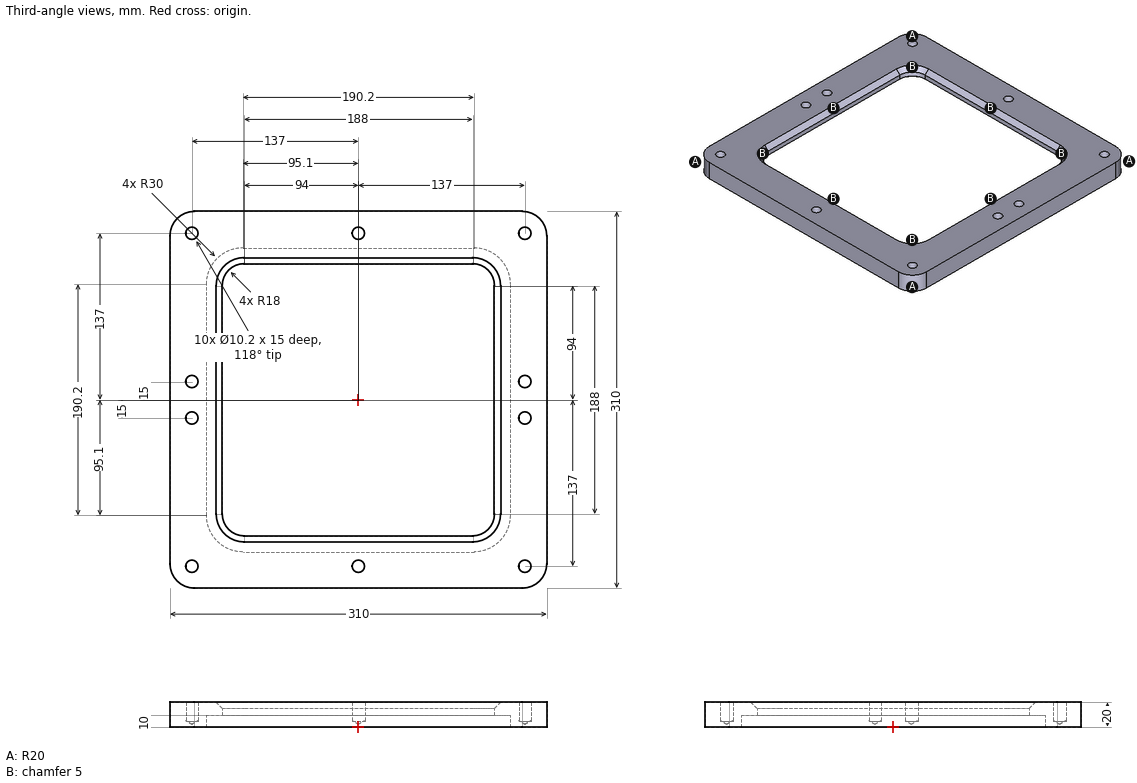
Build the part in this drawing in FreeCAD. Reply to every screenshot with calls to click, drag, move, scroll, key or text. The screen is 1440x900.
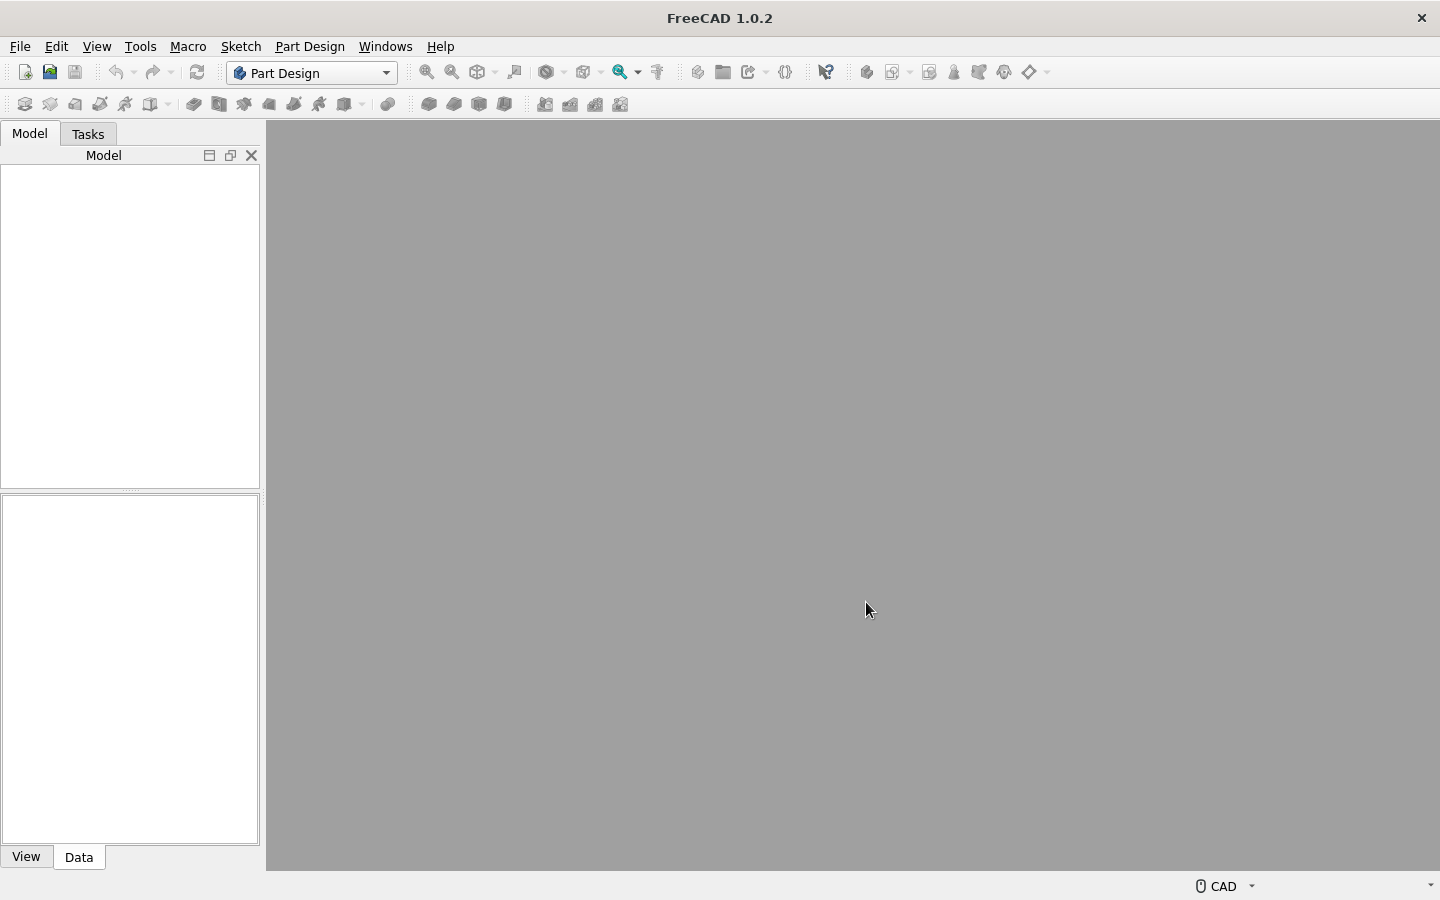
click(25, 72)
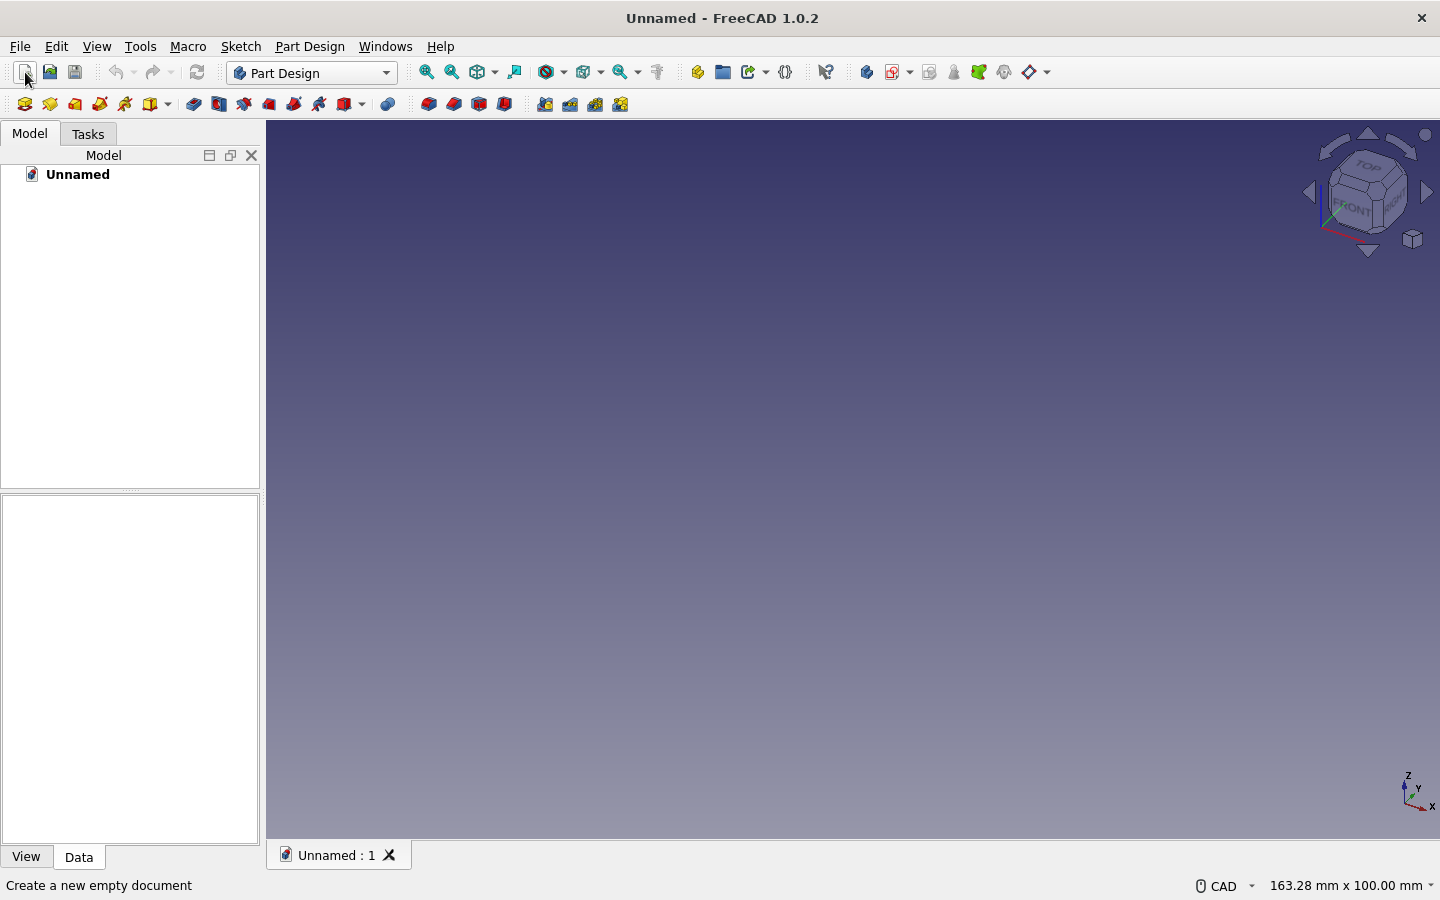
click(892, 72)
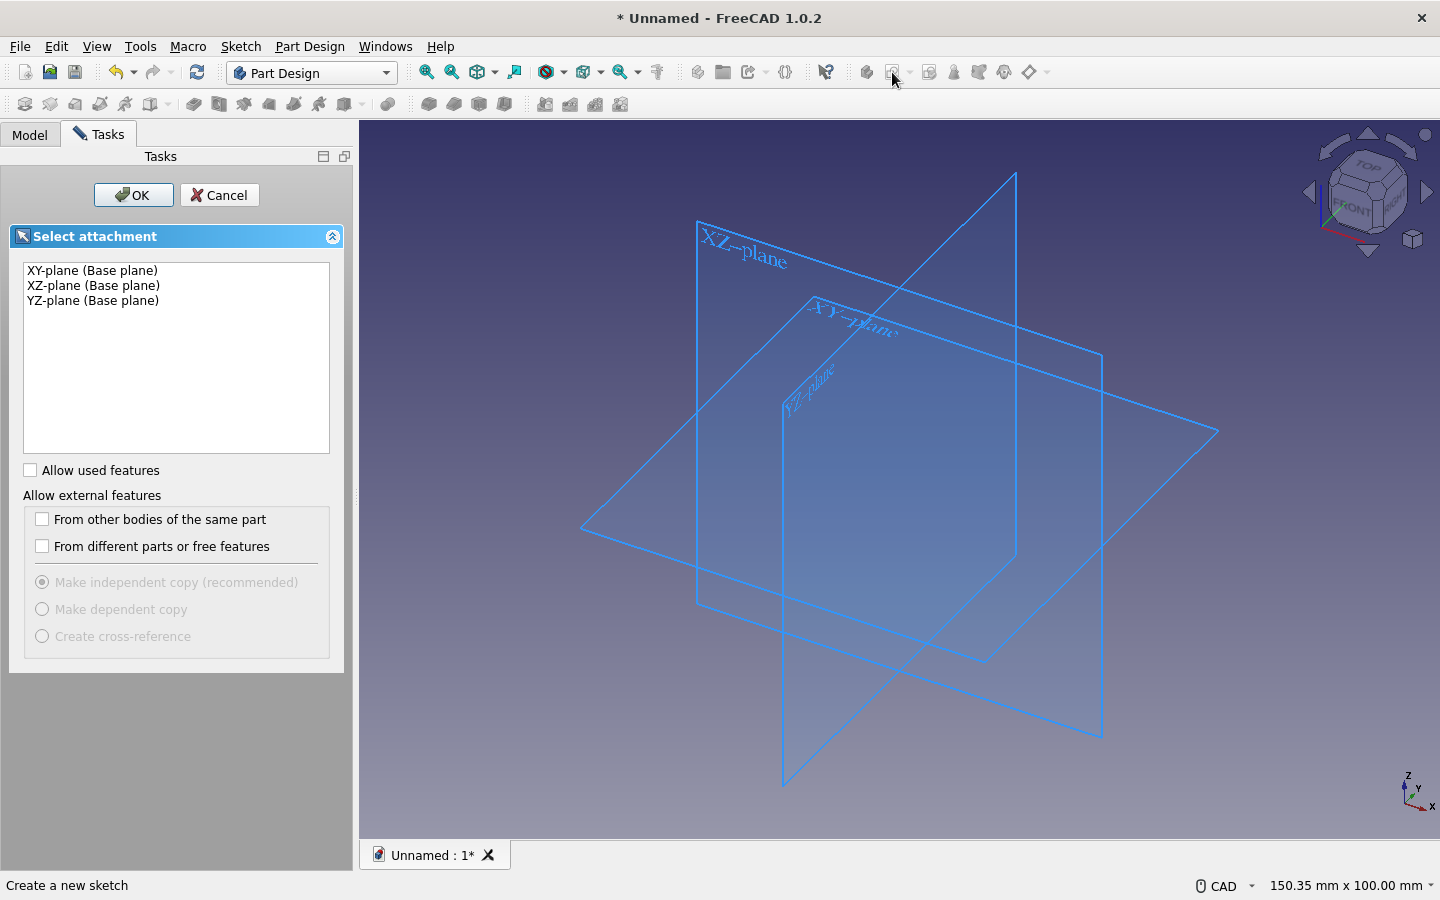
click(84, 270)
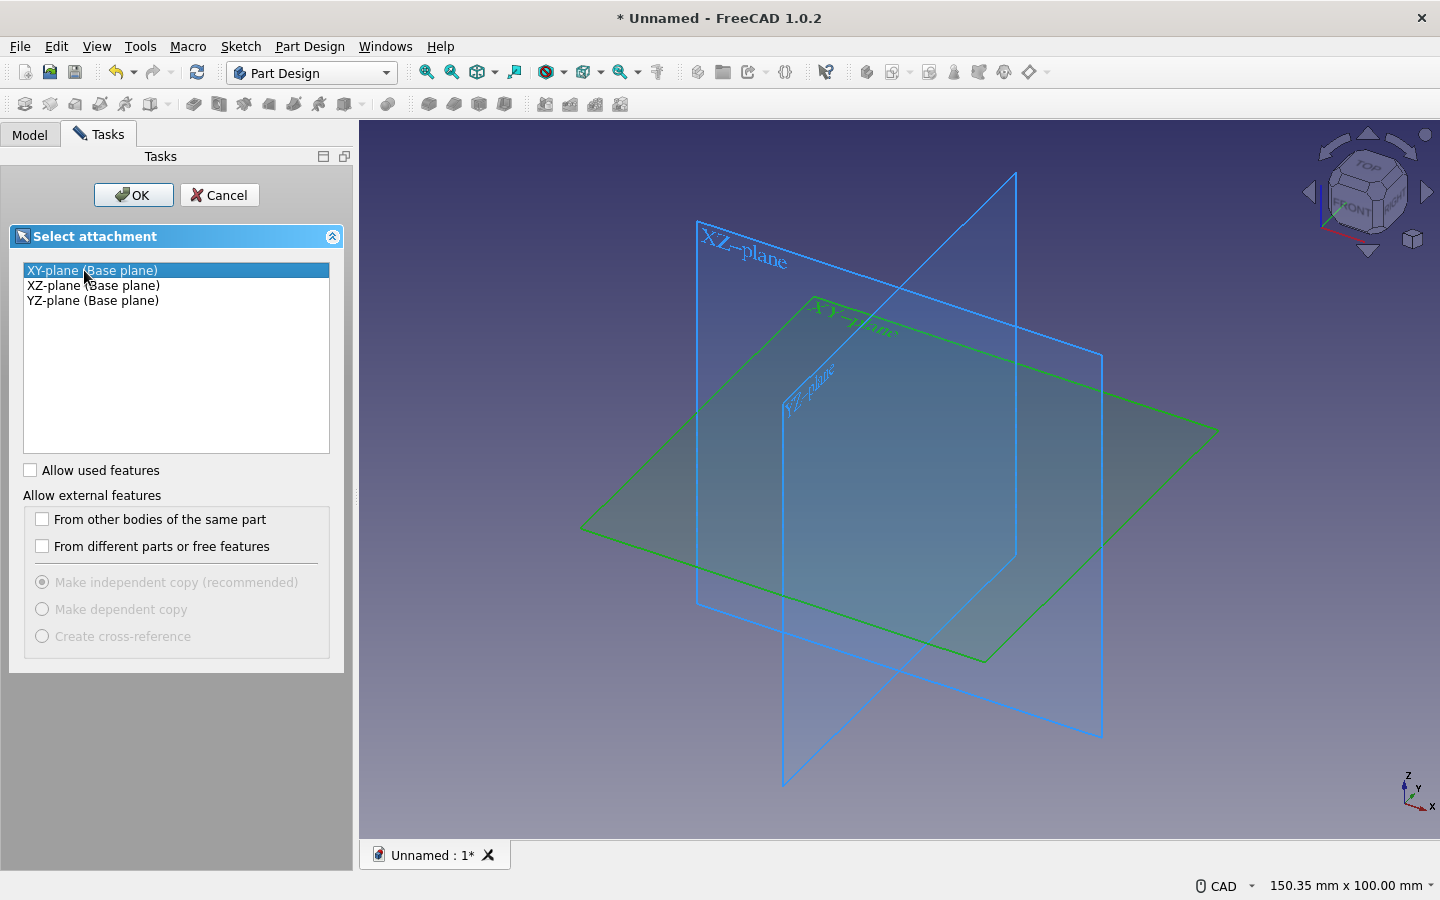
click(134, 195)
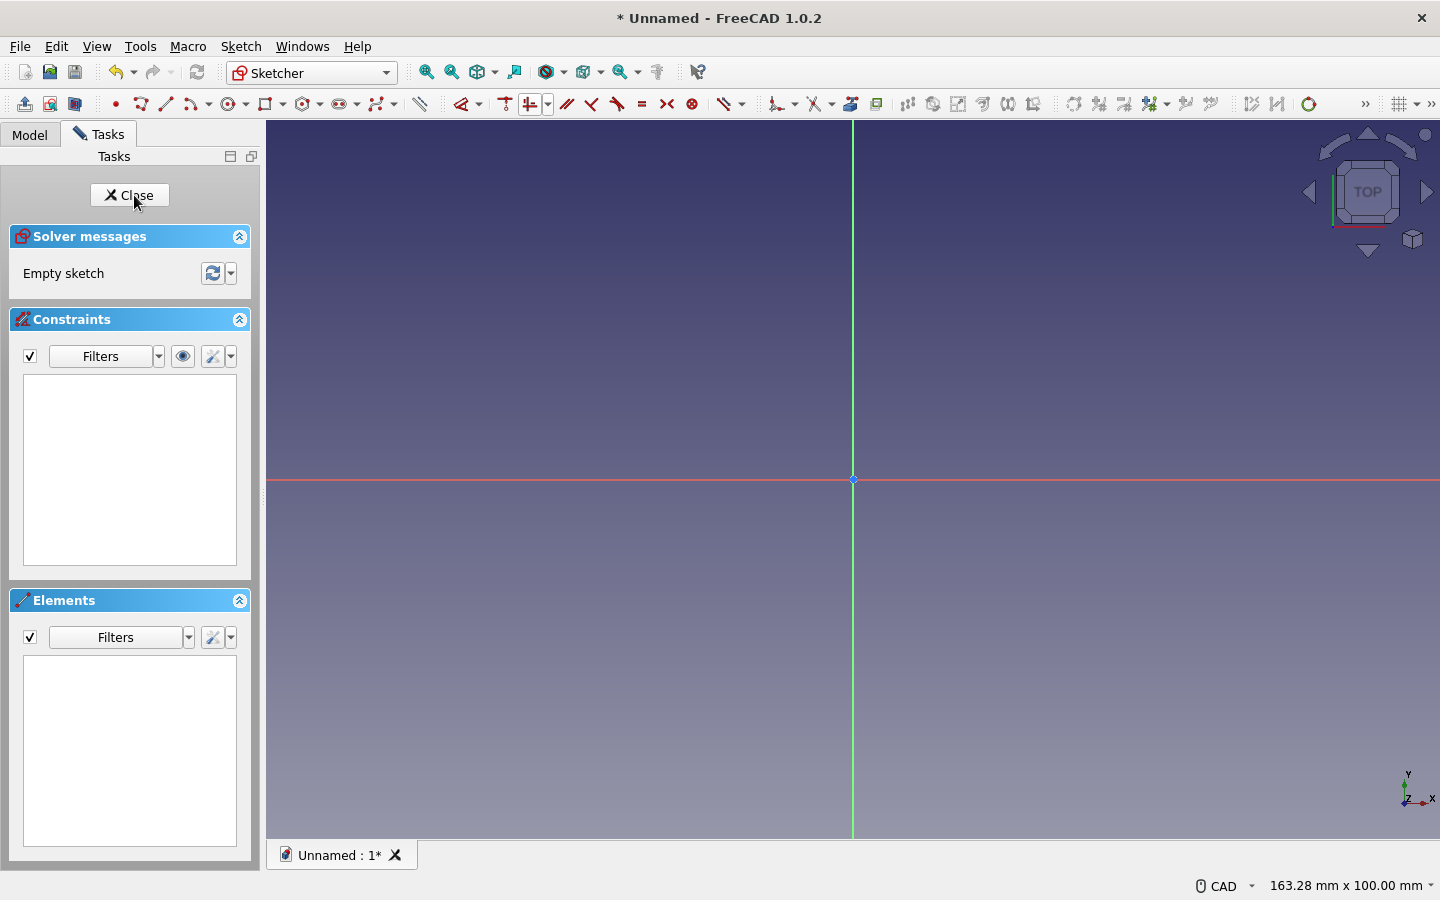
scroll(767, 480, down, 8)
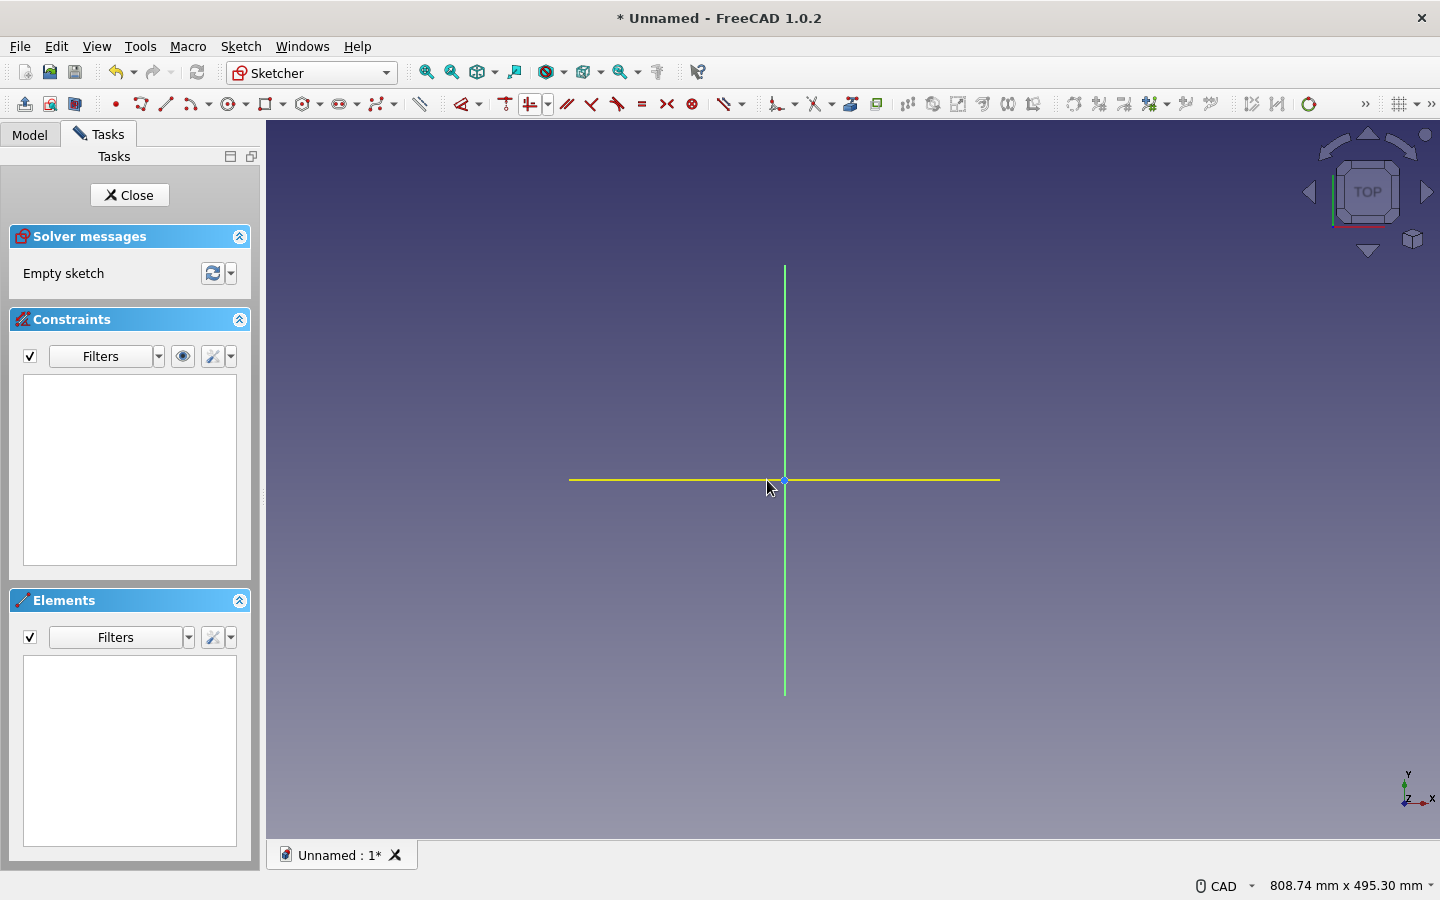
key(g)
key(v)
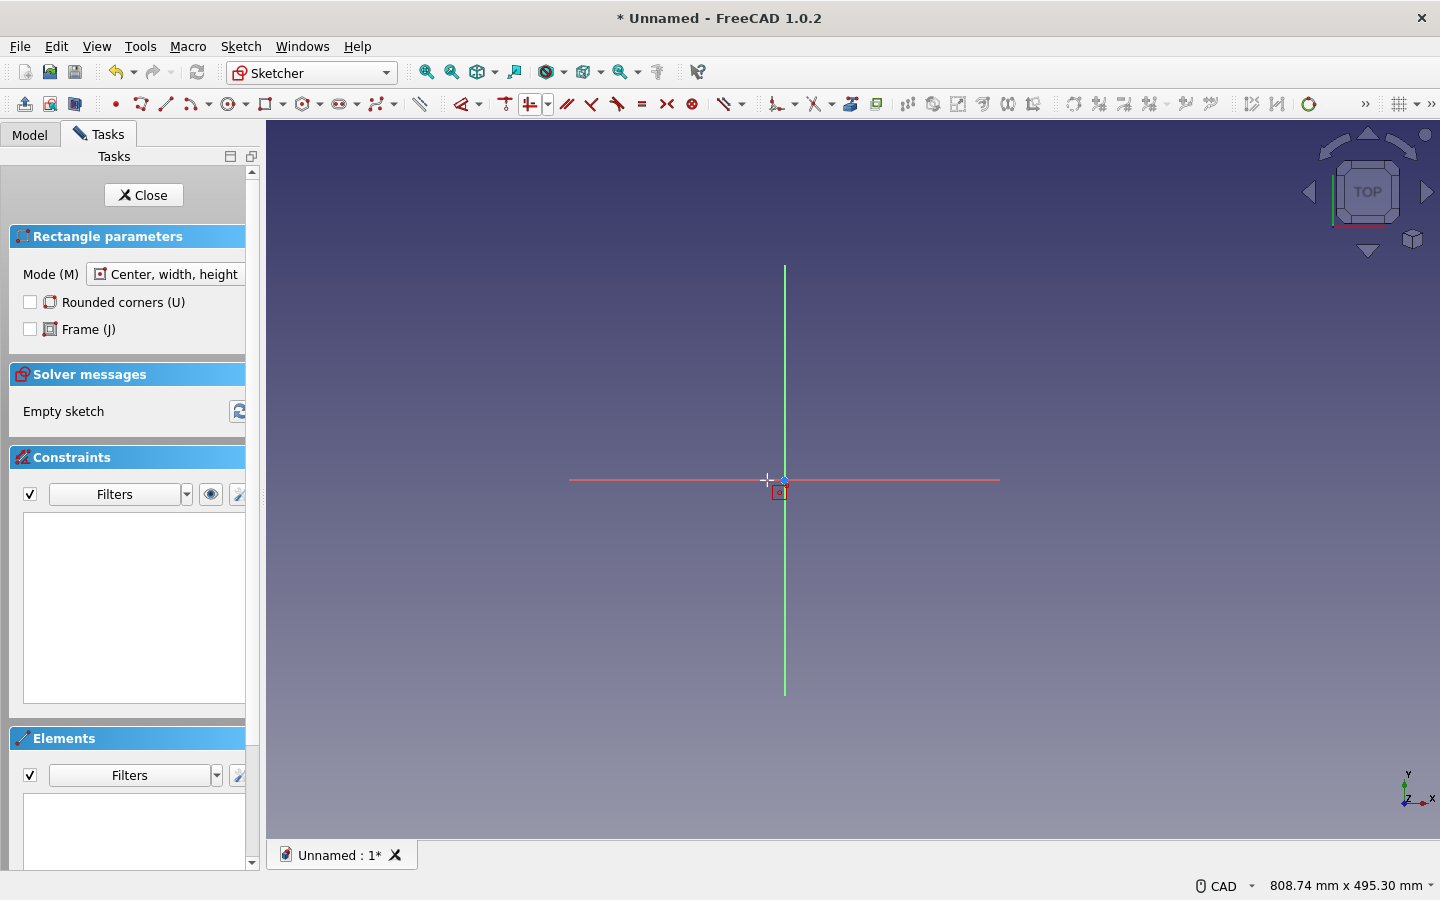
click(785, 480)
click(1010, 255)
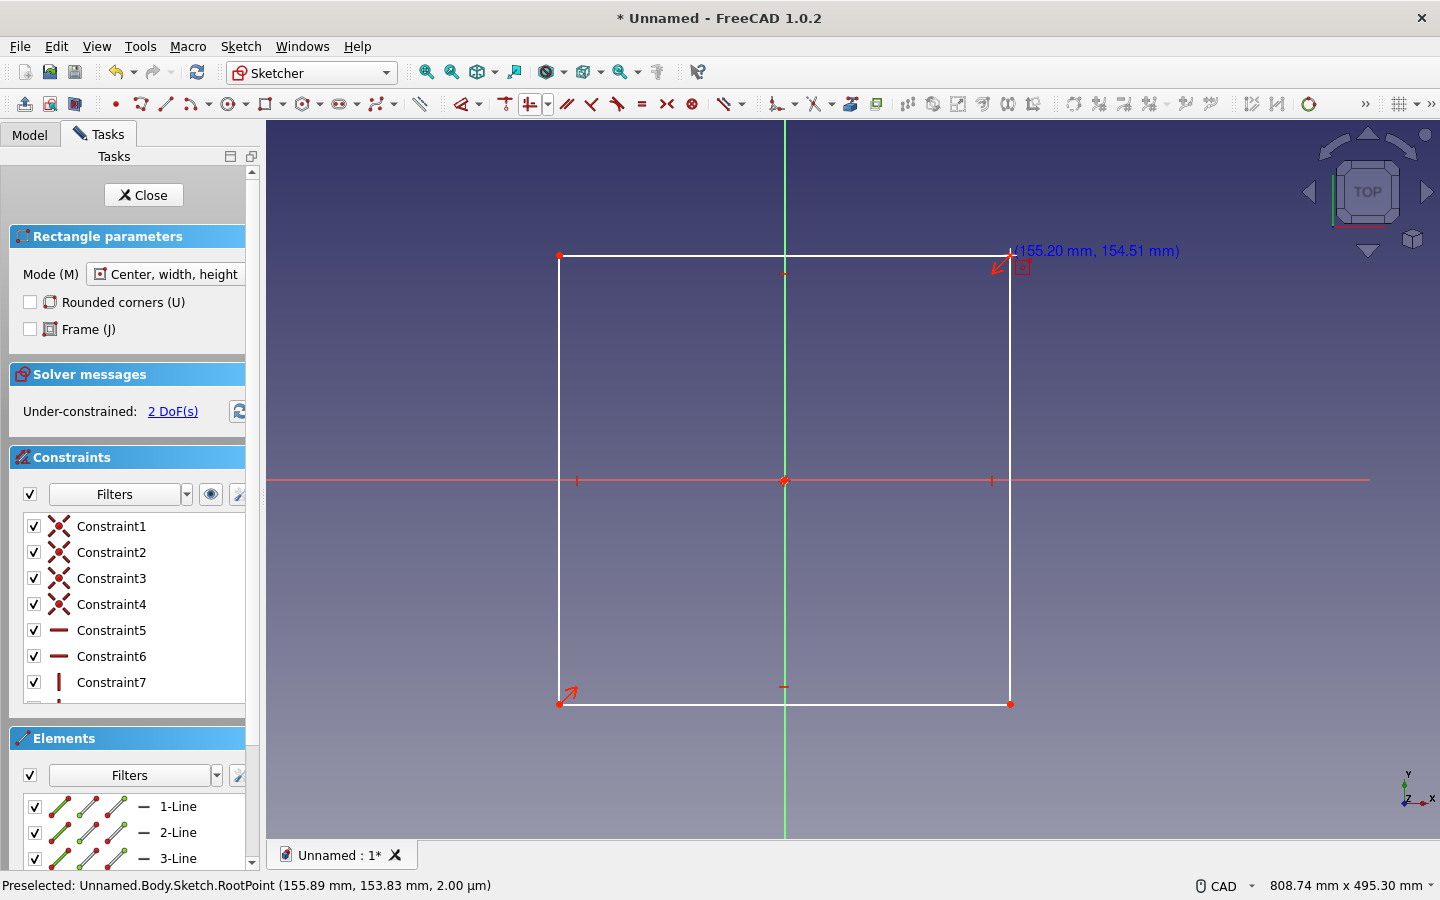
click(166, 104)